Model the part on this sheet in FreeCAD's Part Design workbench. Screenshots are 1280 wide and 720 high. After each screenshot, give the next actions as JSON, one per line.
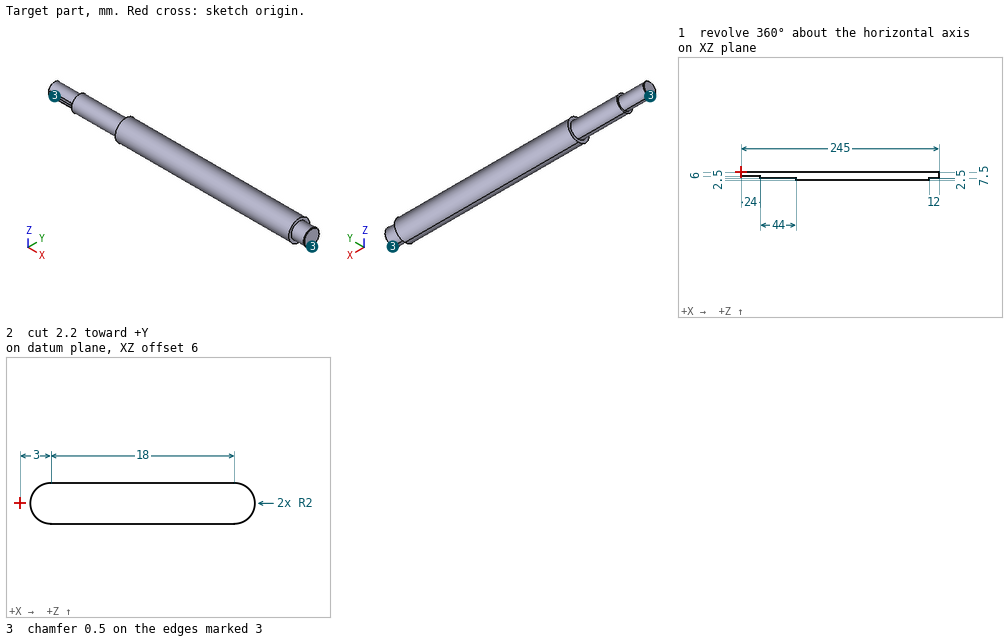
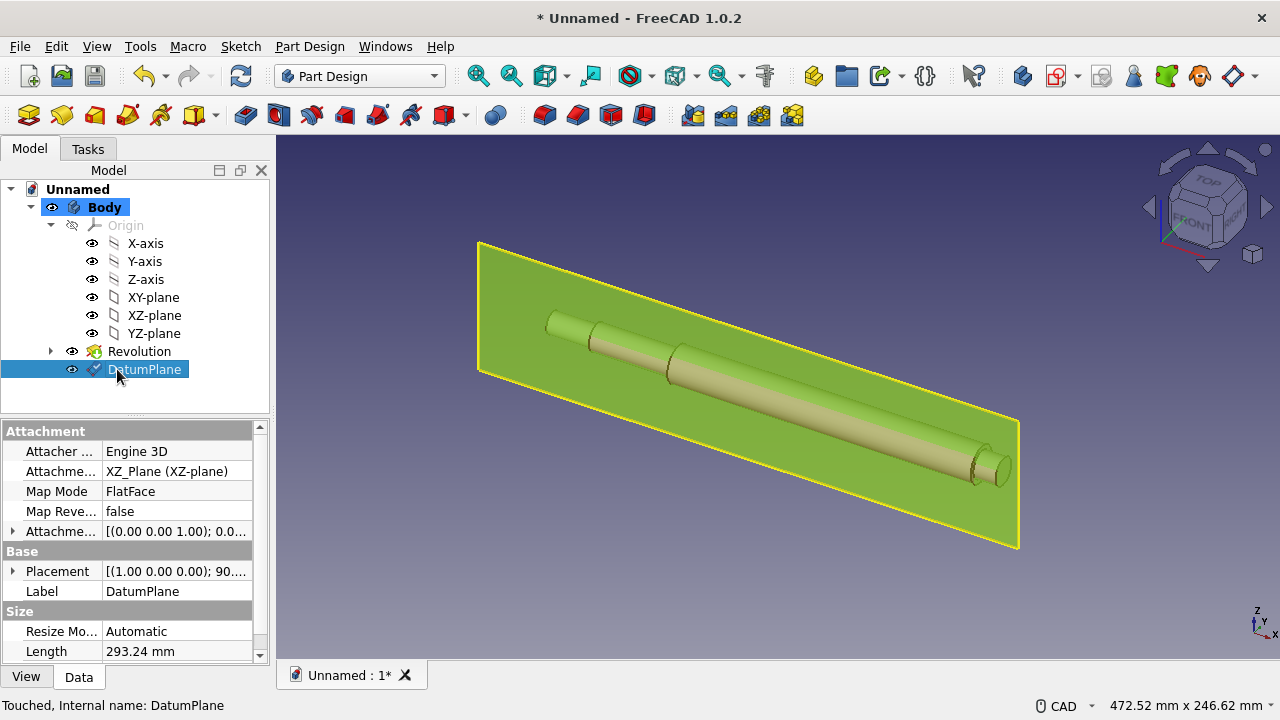
{"action": "left_click", "coordinate": [1056, 76]}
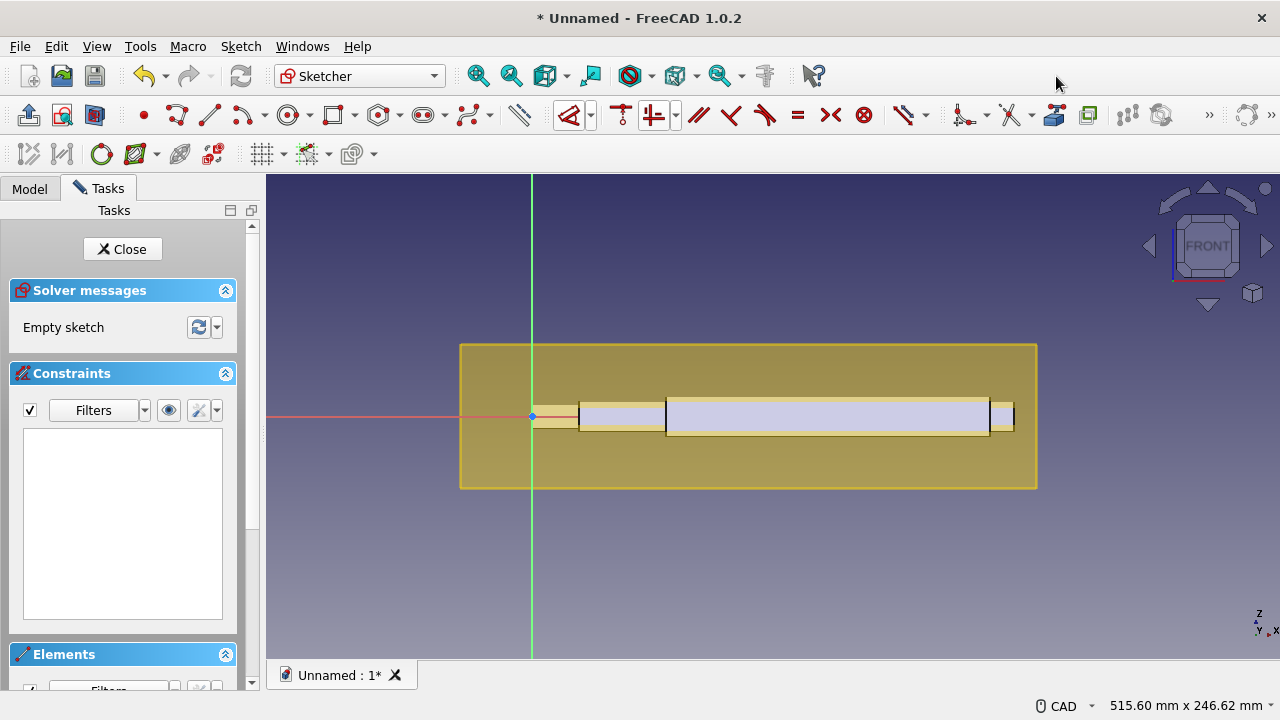
{"action": "left_click", "coordinate": [95, 116]}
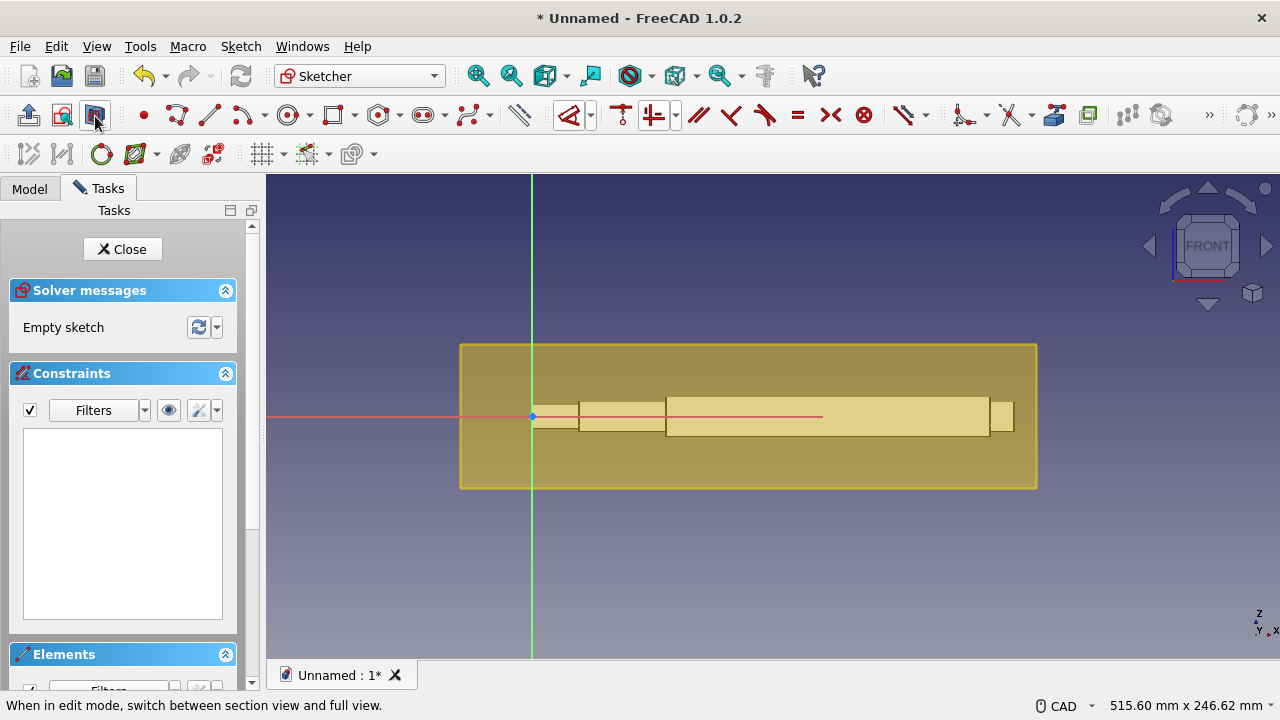
{"action": "scroll", "coordinate": [543, 416], "scroll_direction": "up", "scroll_amount": 13}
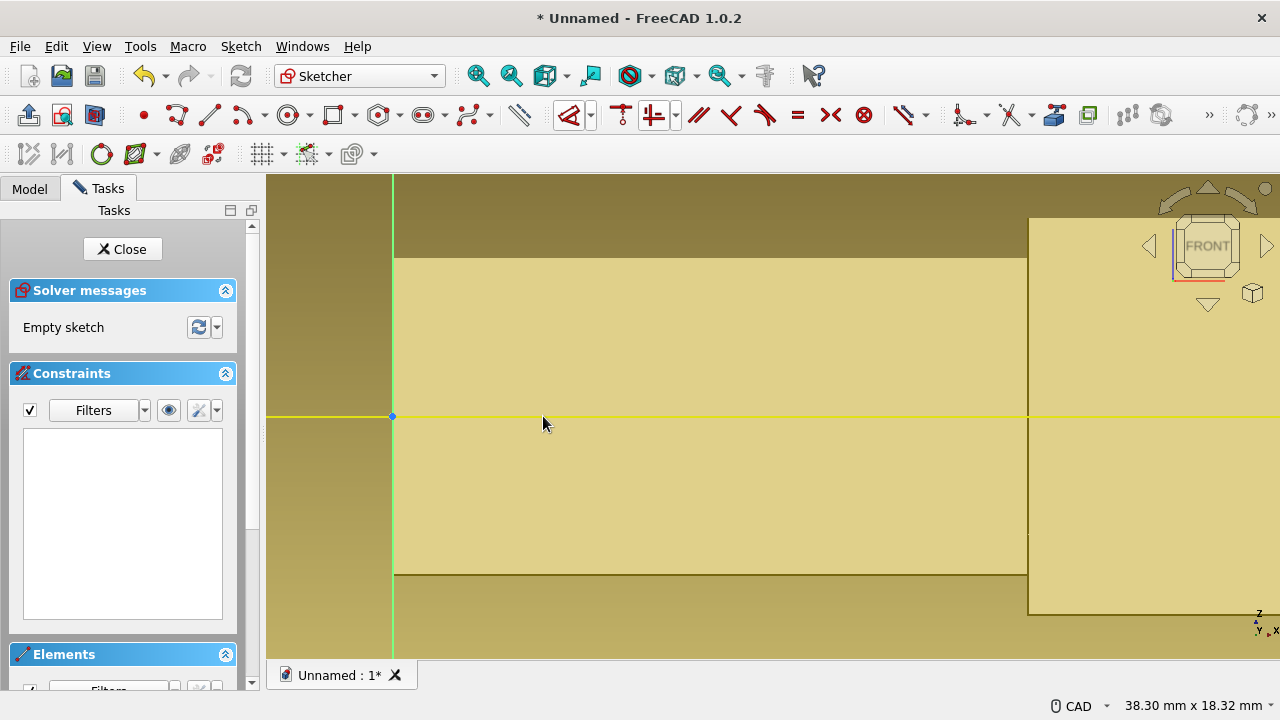
{"action": "left_click", "coordinate": [422, 116]}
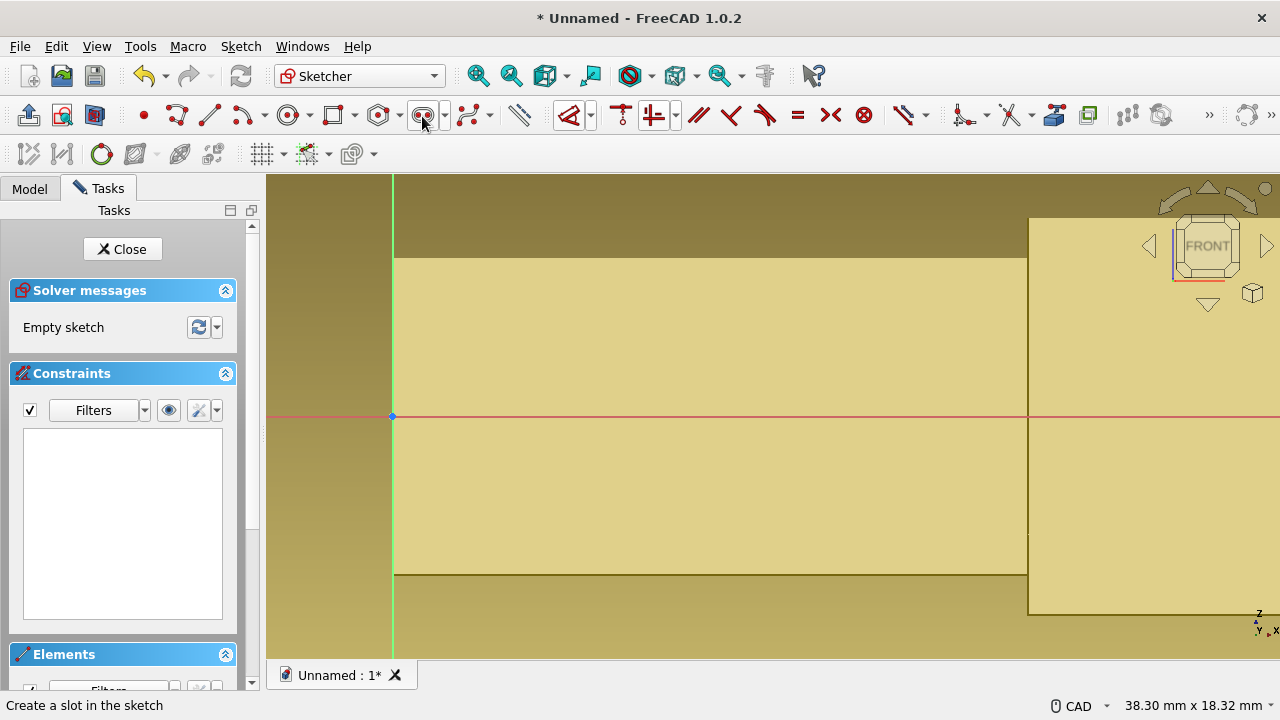
{"action": "left_click", "coordinate": [472, 416]}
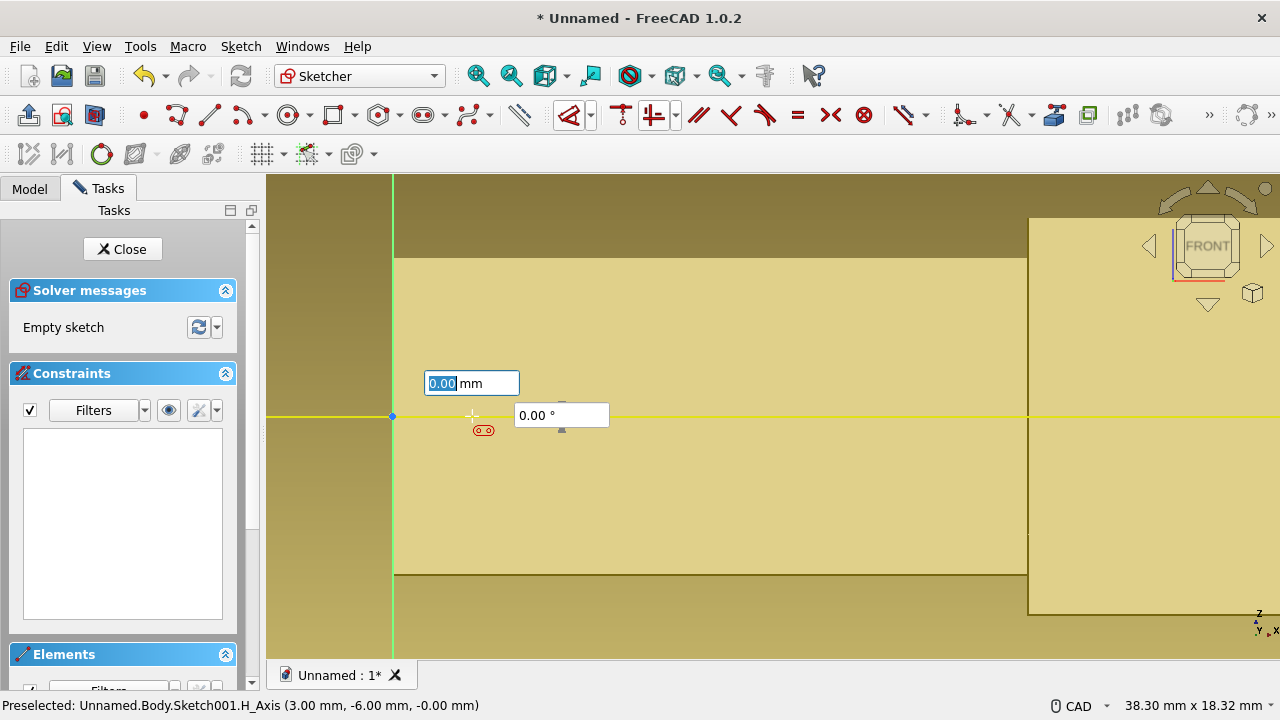
{"action": "left_click", "coordinate": [949, 407]}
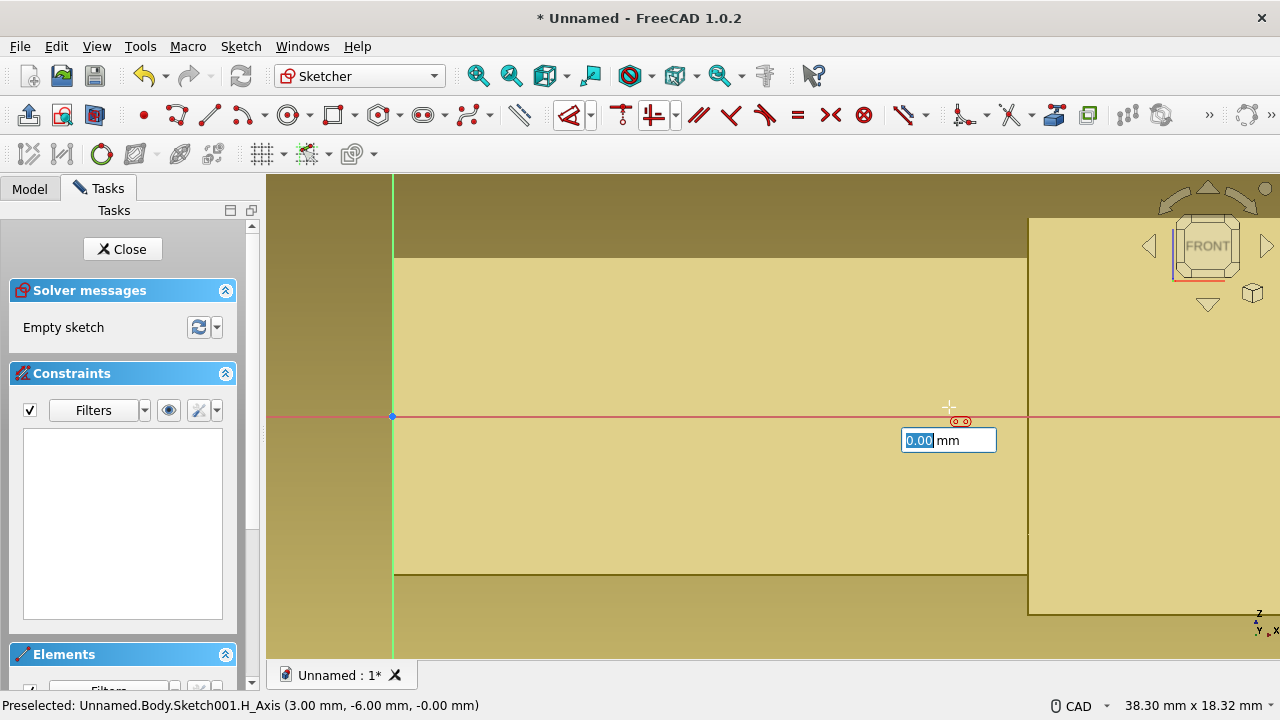
{"action": "left_click", "coordinate": [710, 469]}
{"action": "key", "text": "Escape"}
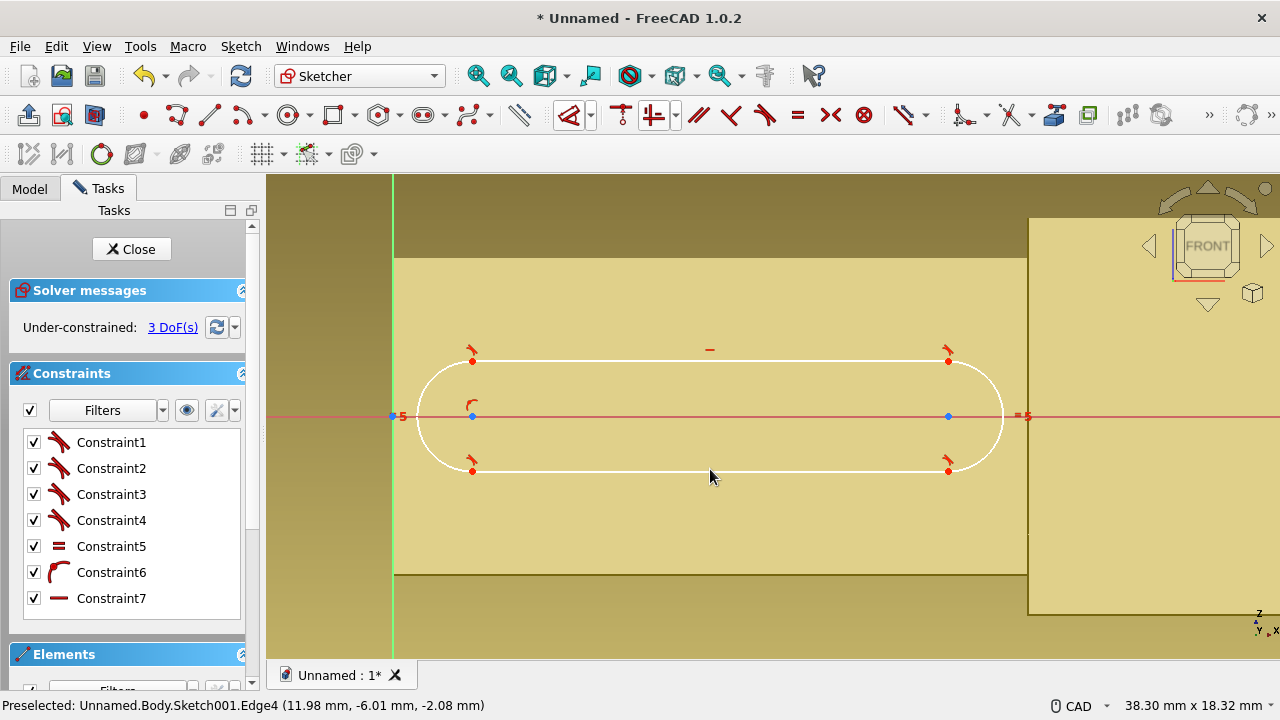
{"action": "left_click", "coordinate": [428, 384]}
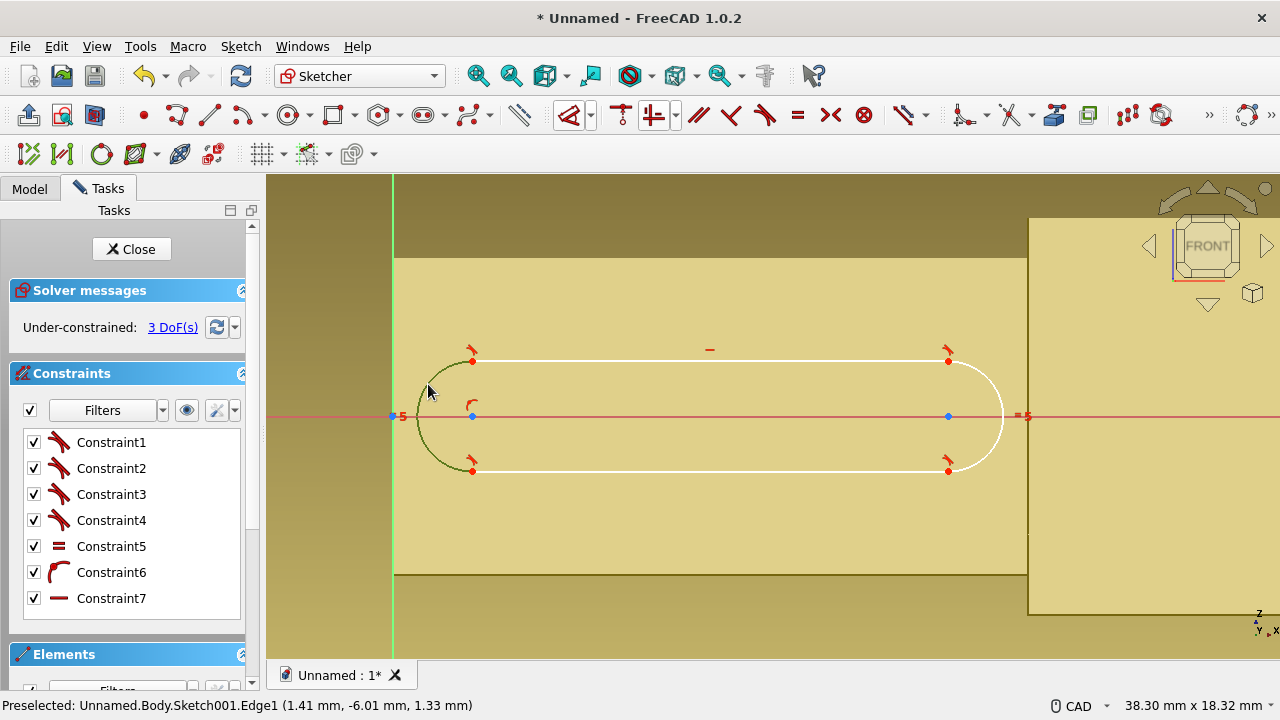
{"action": "left_click", "coordinate": [590, 116]}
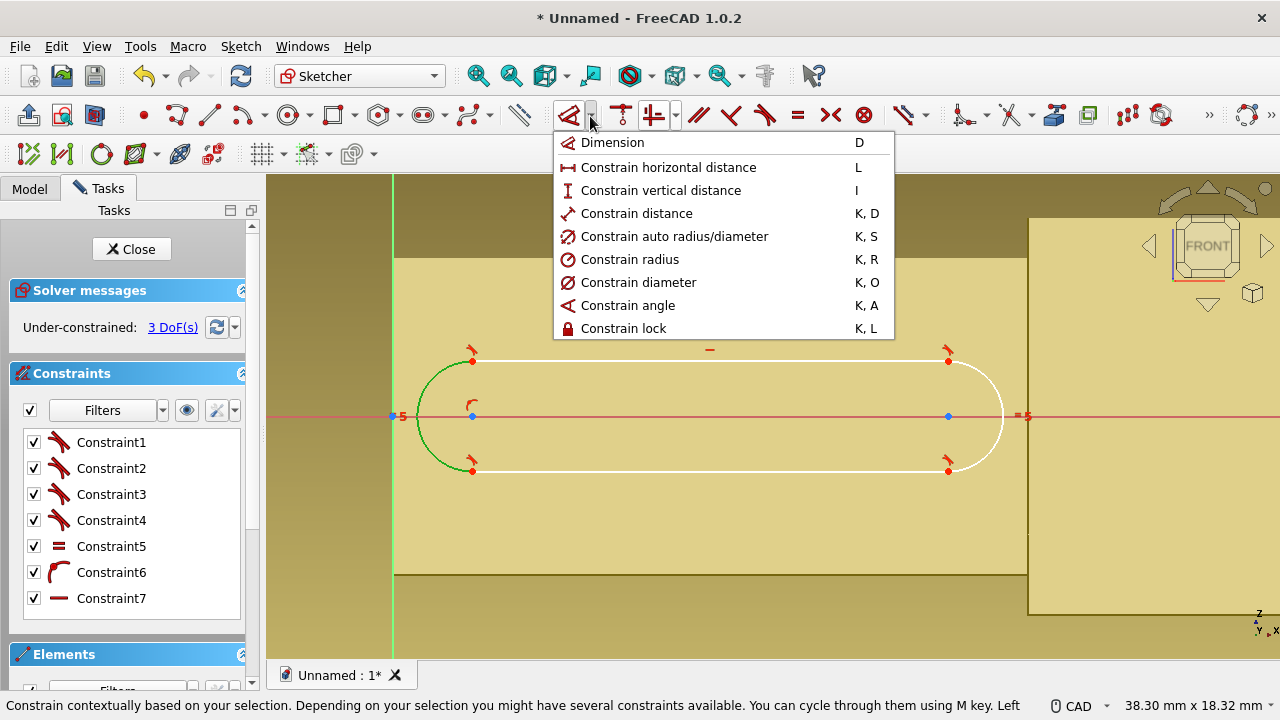
{"action": "left_click", "coordinate": [724, 260]}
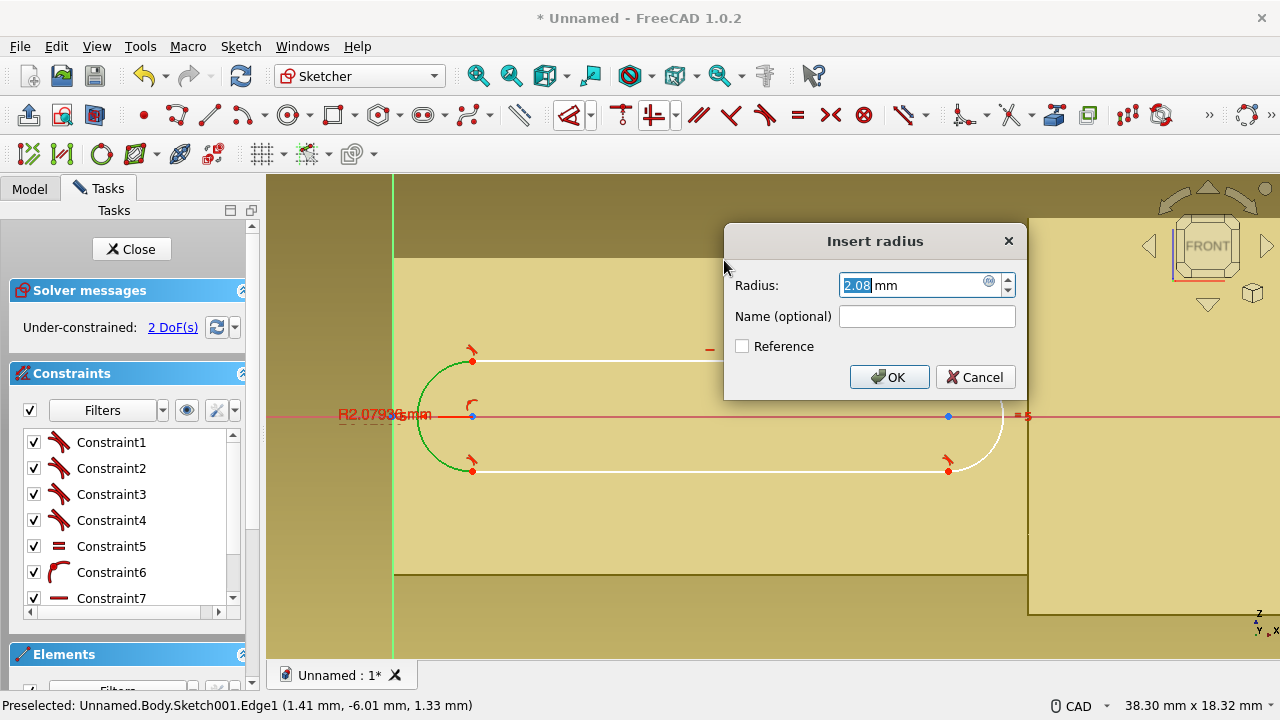
{"action": "type", "text": "2"}
{"action": "key", "text": "Return"}